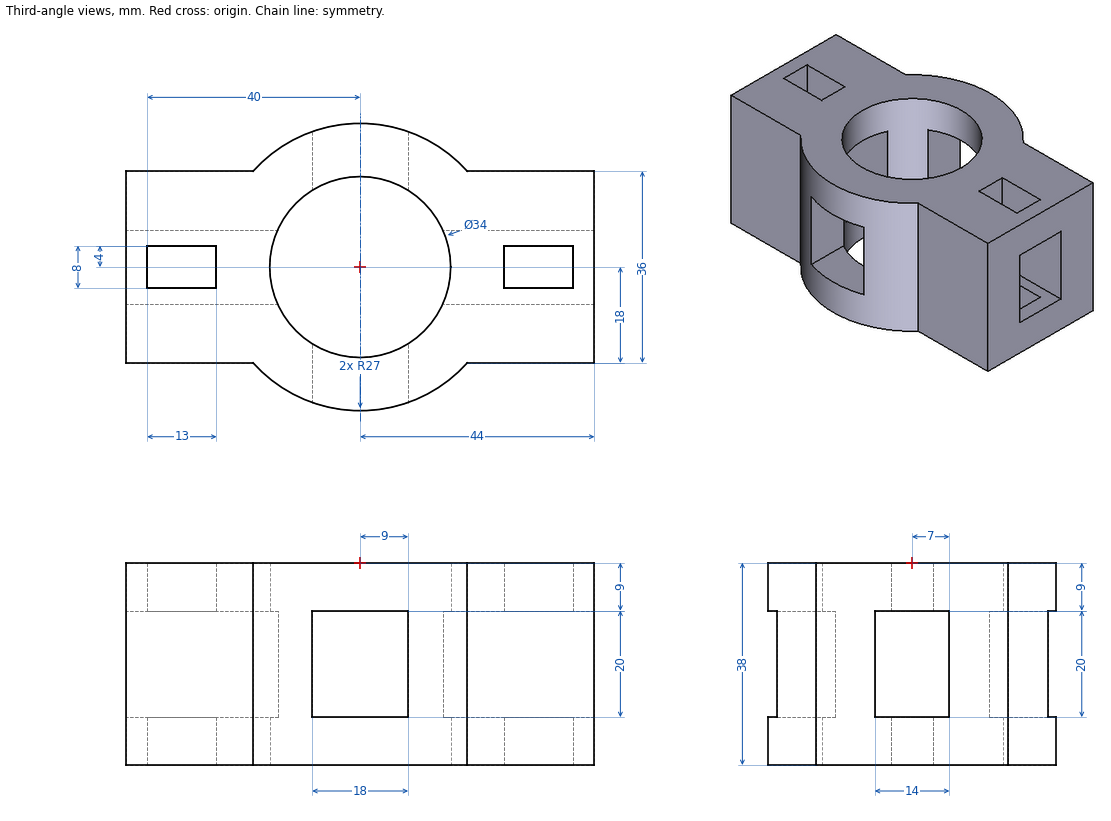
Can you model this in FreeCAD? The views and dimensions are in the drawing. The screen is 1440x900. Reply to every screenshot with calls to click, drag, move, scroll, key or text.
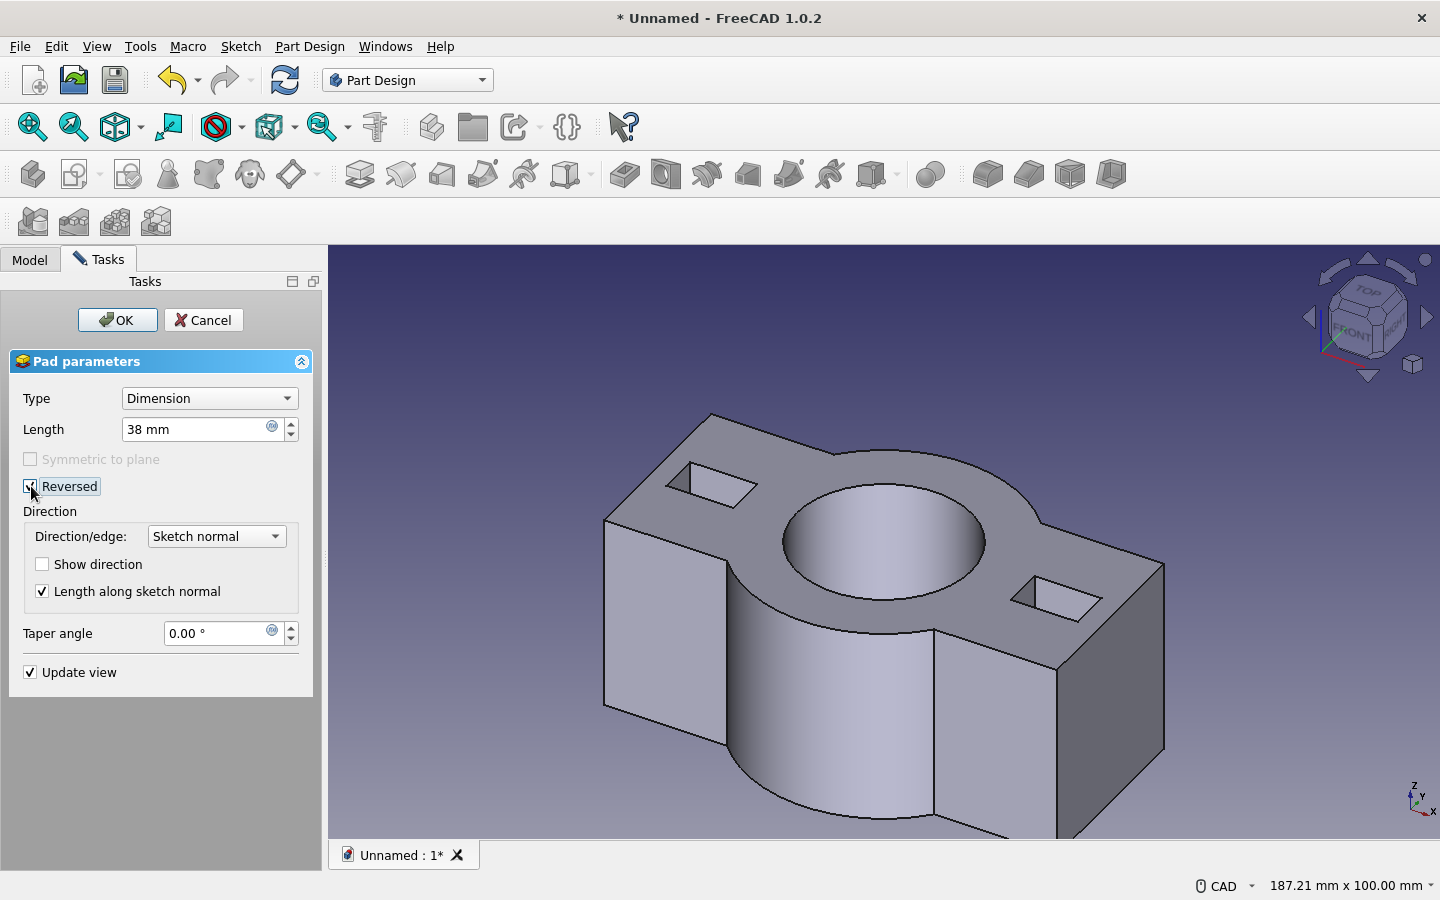
click(118, 320)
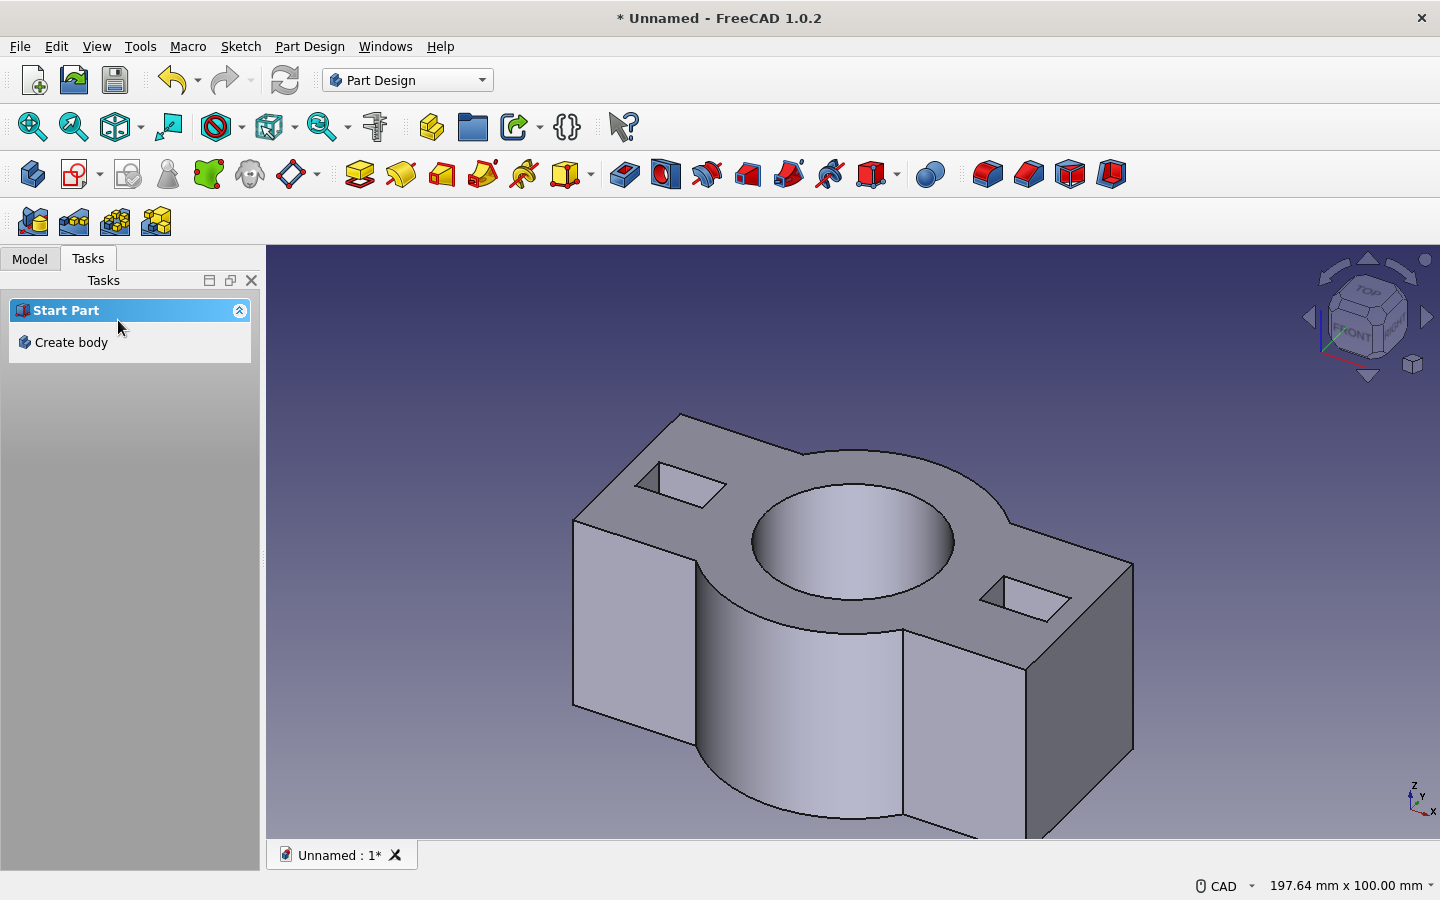
click(33, 128)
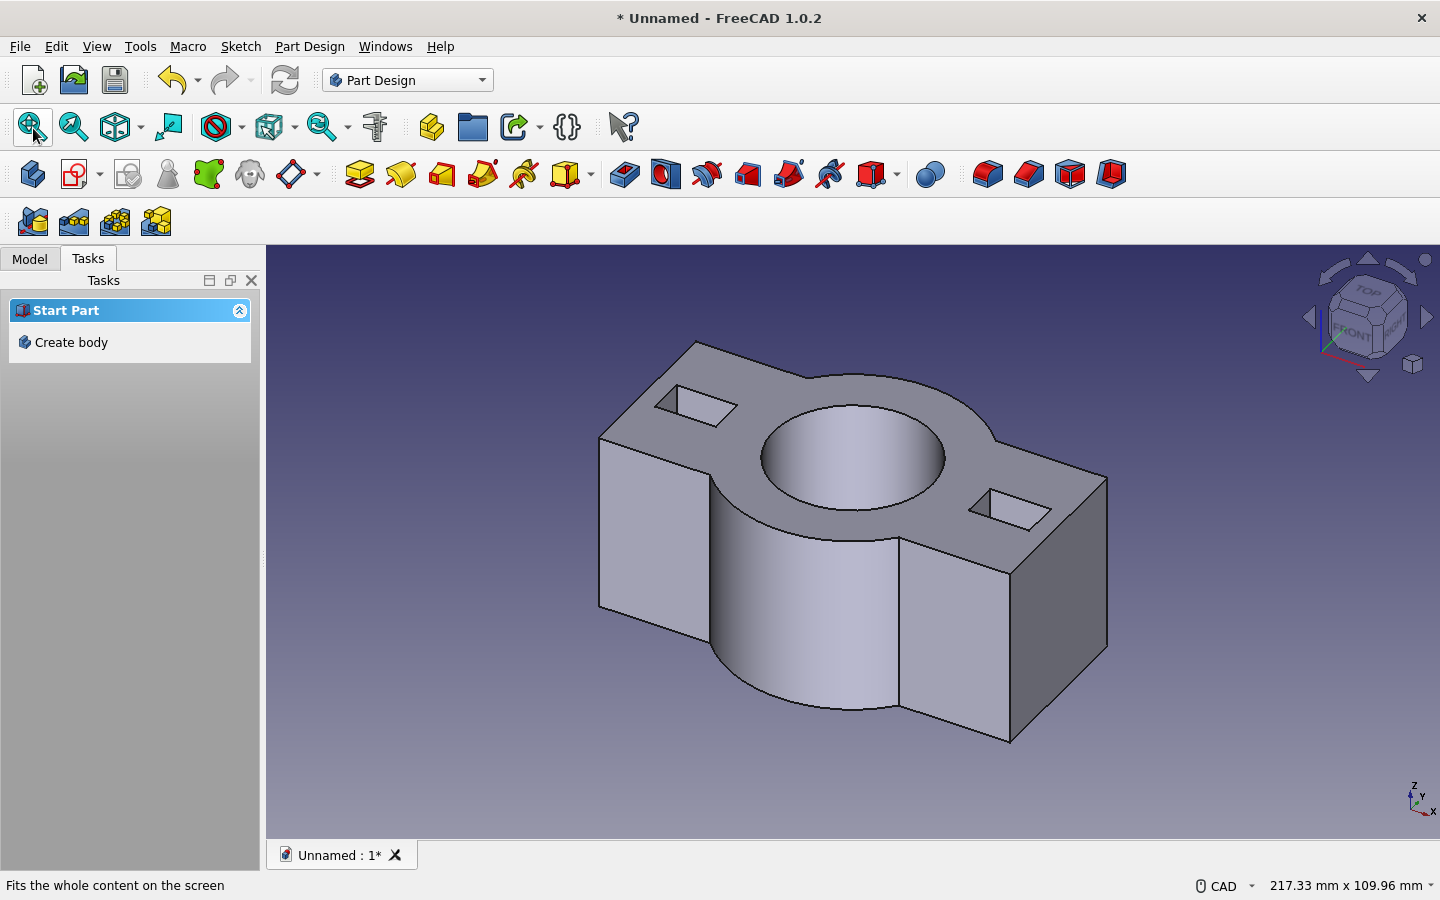
key(6)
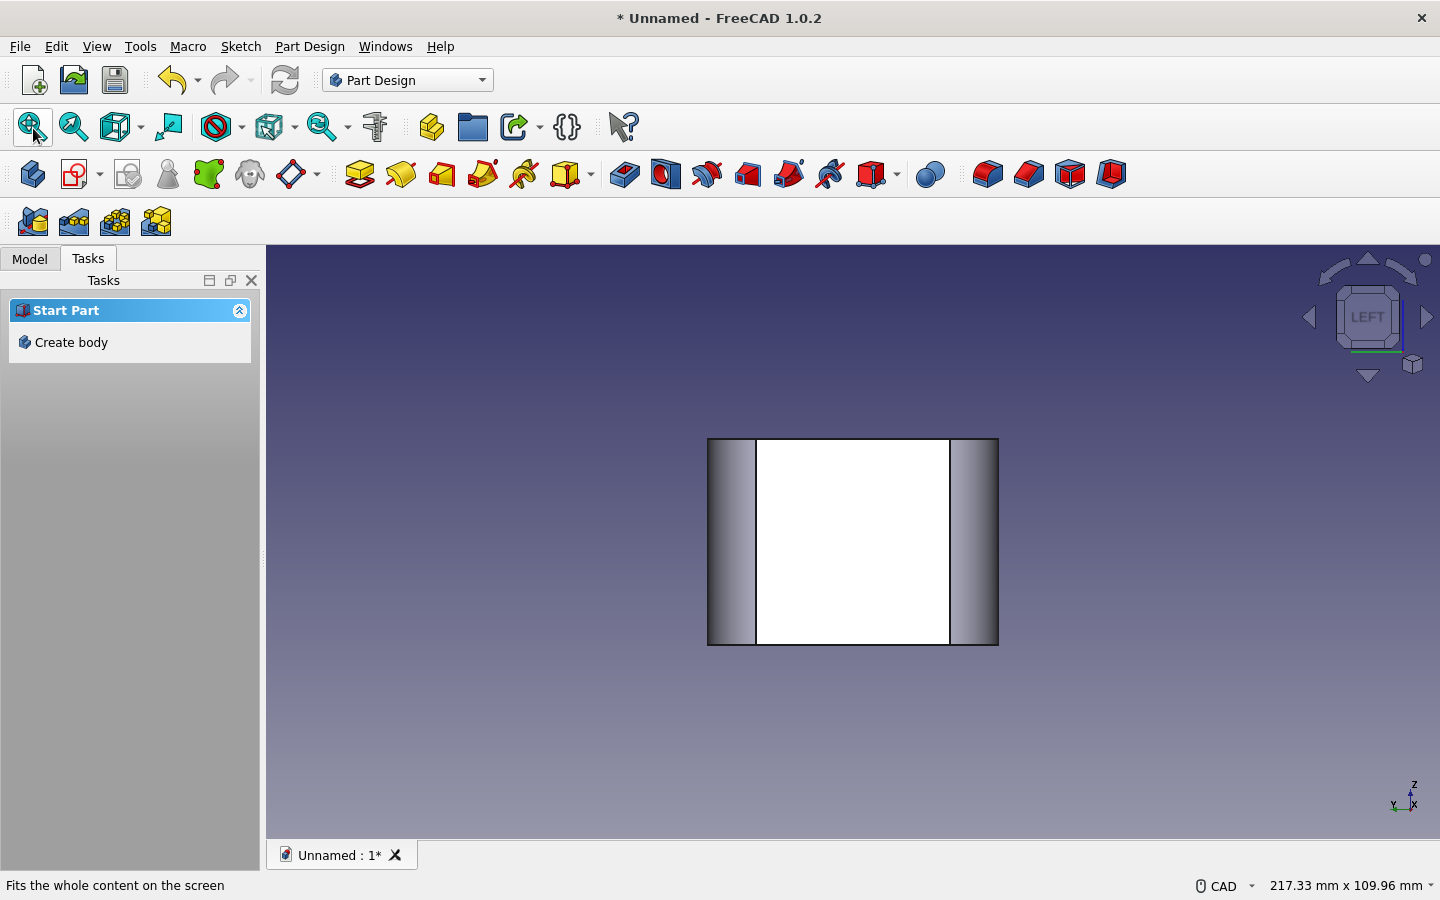
click(33, 128)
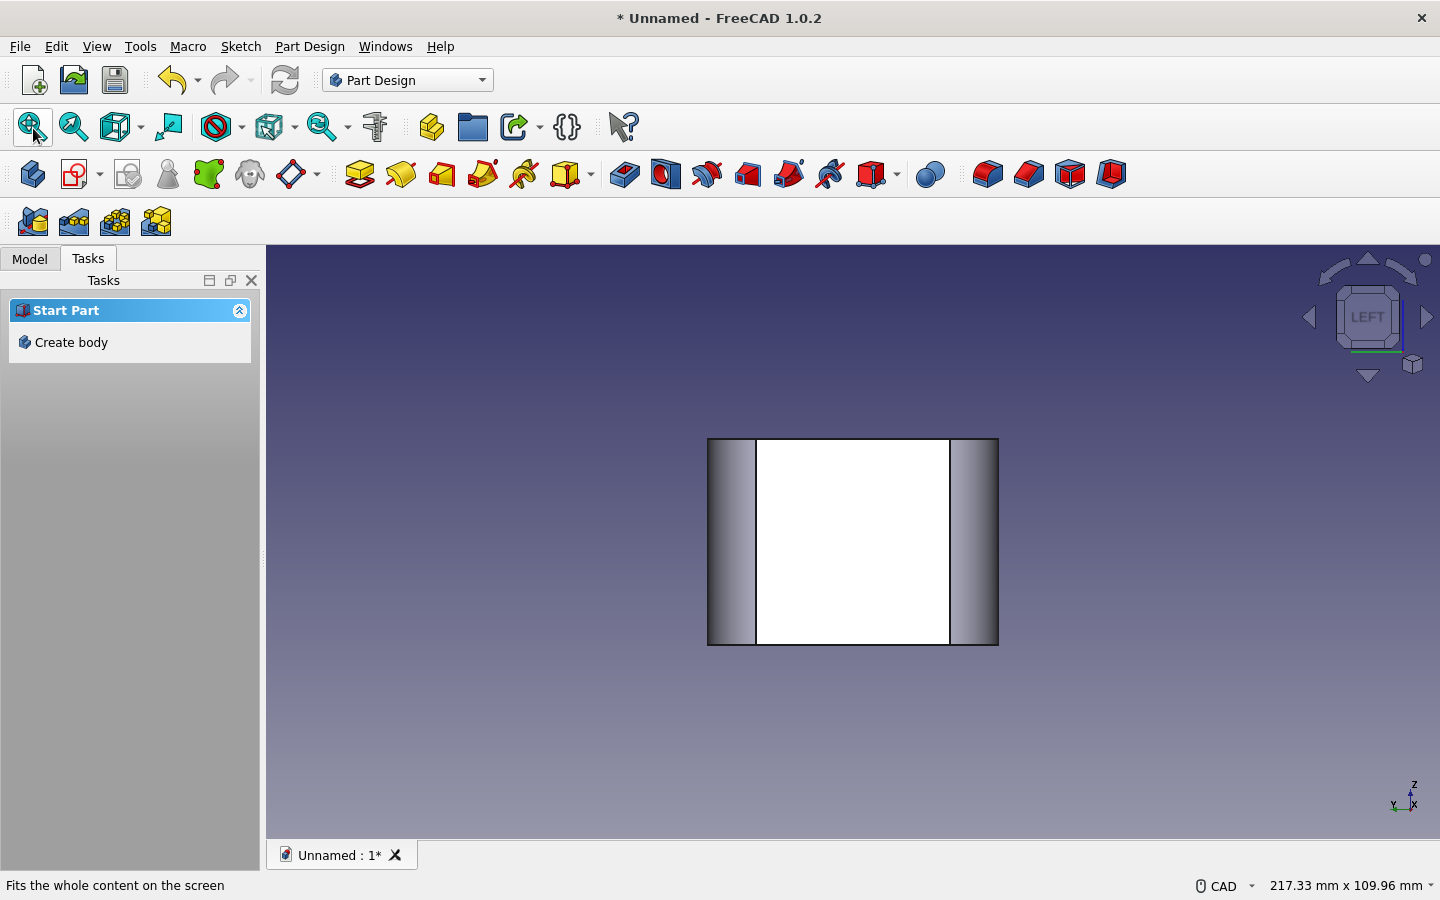
click(853, 541)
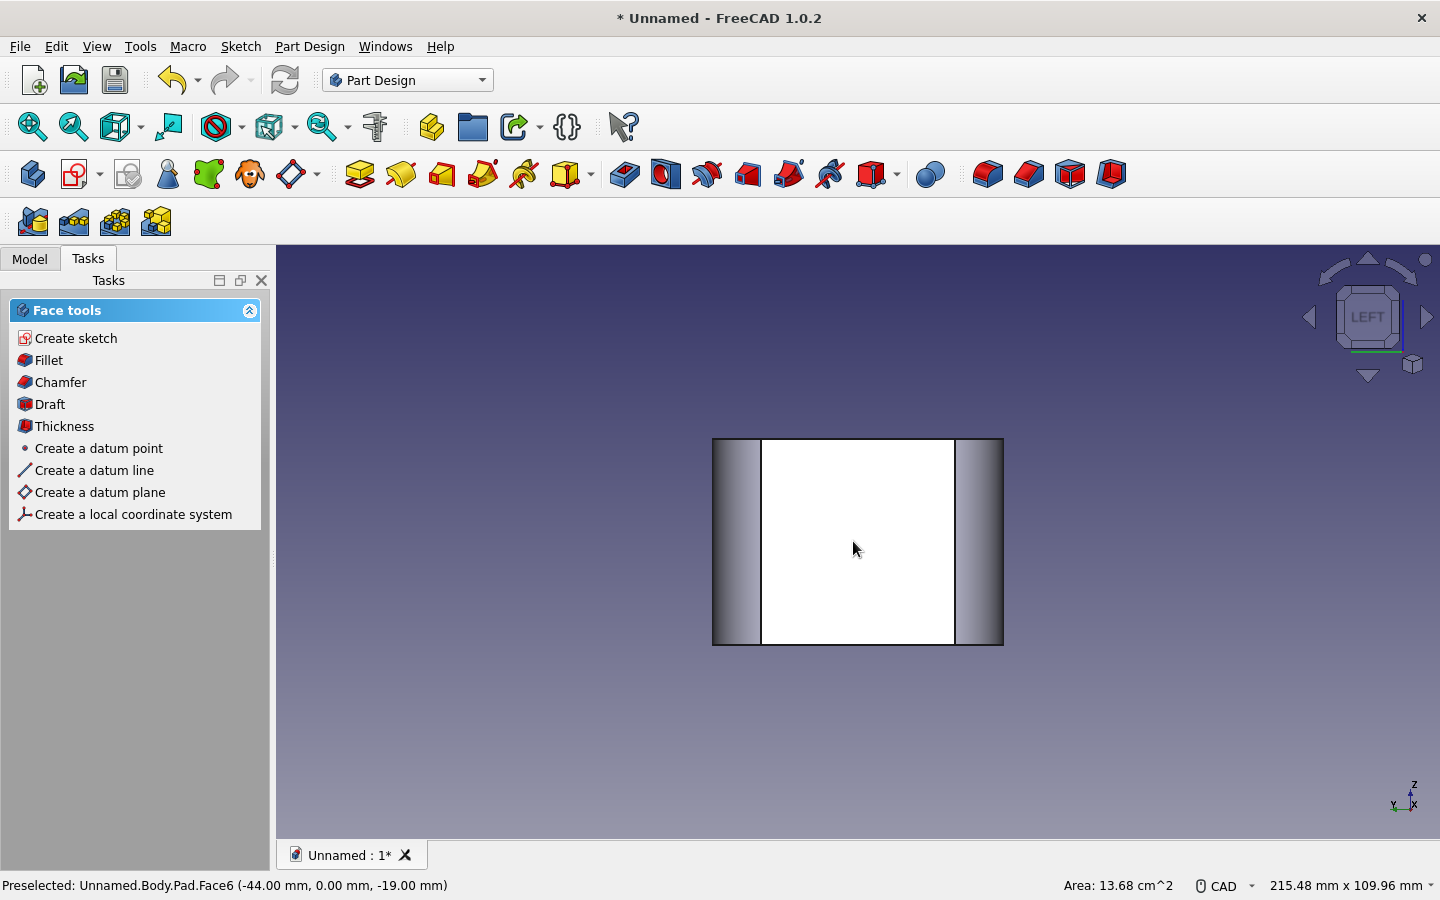
click(74, 174)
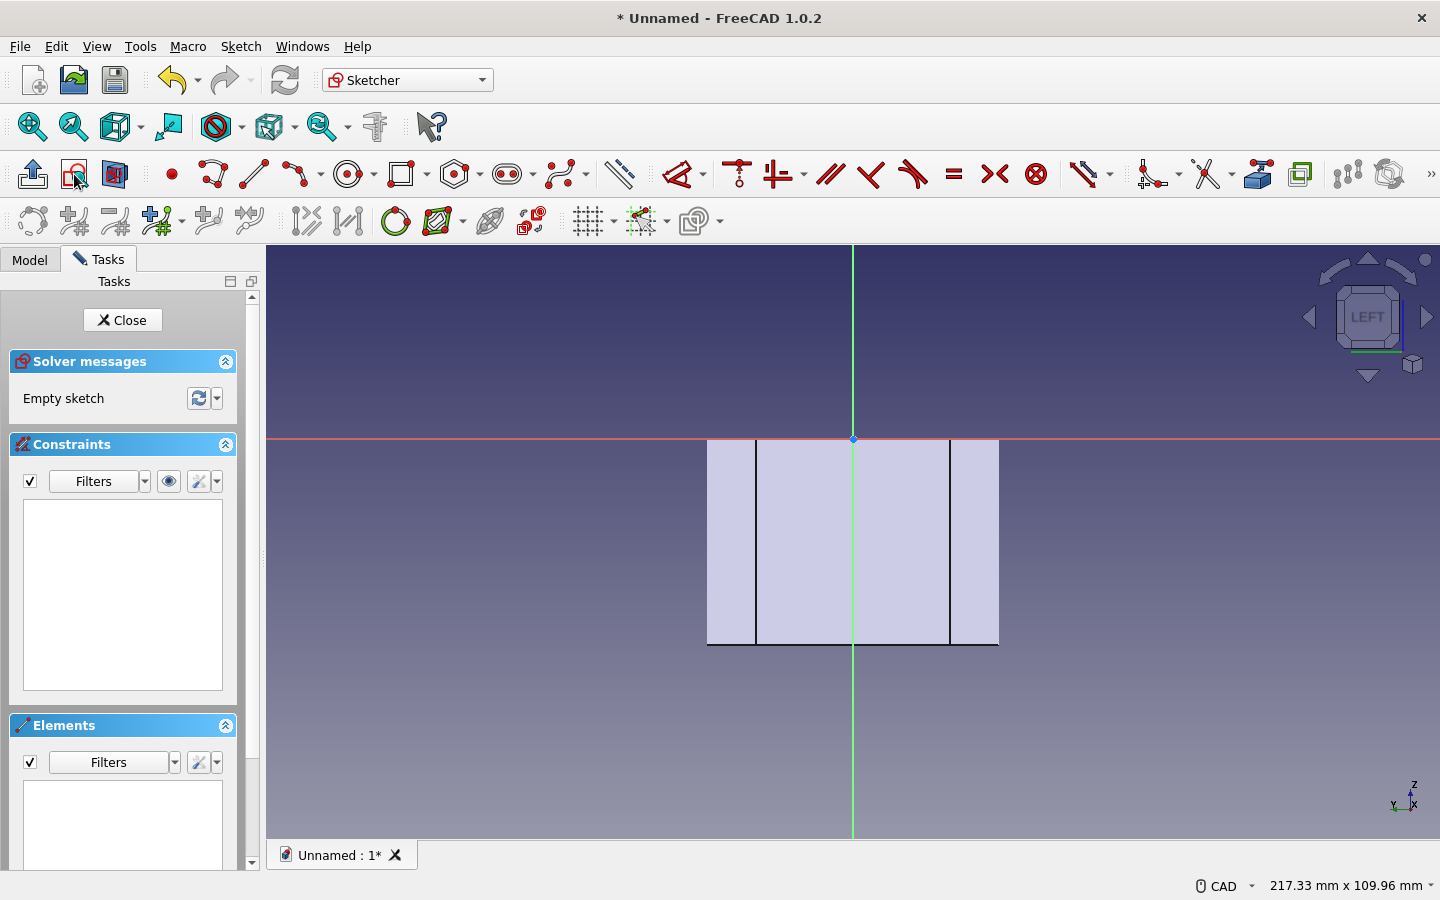
scroll(909, 498, up, 4)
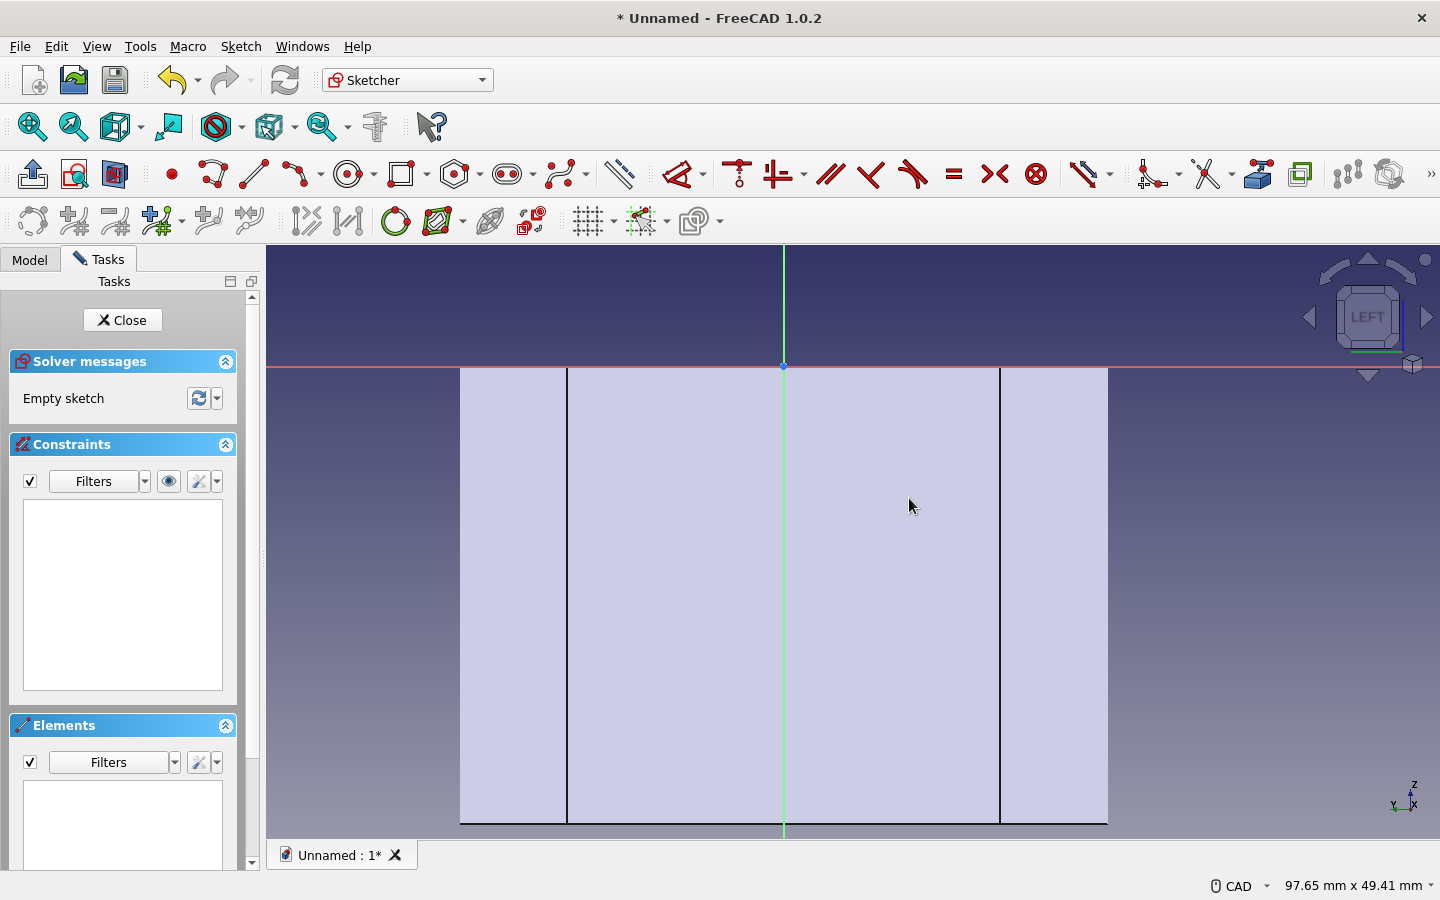
click(400, 174)